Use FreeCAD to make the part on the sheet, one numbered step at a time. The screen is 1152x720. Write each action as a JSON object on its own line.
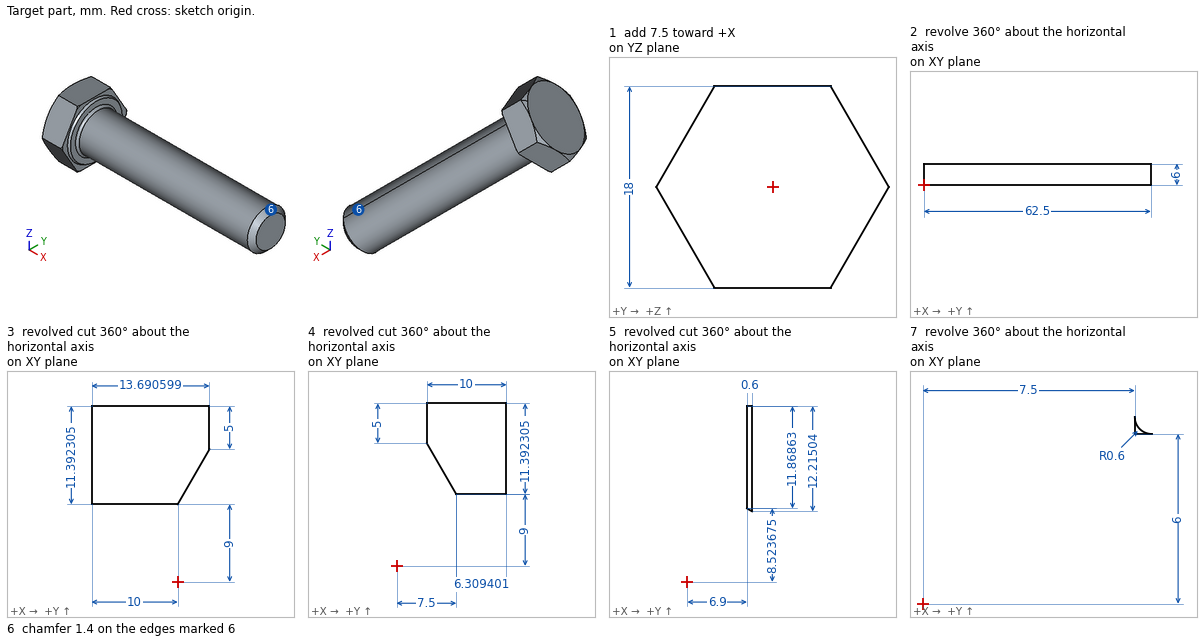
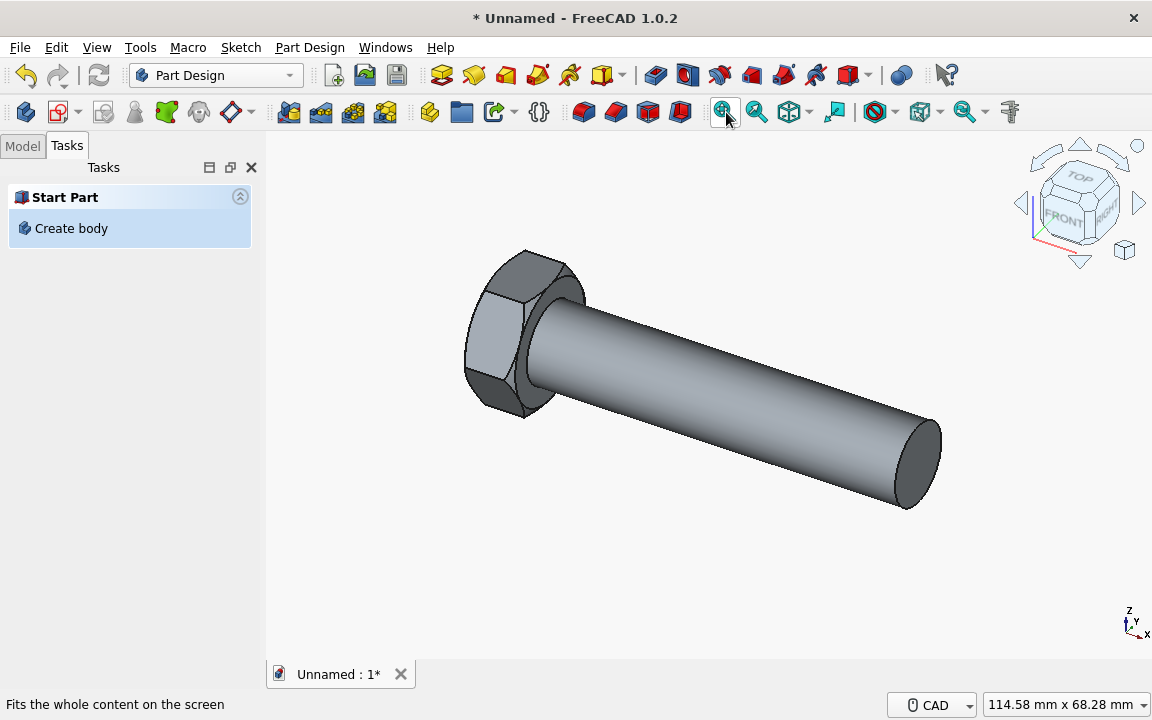
{"action": "left_click", "coordinate": [58, 112]}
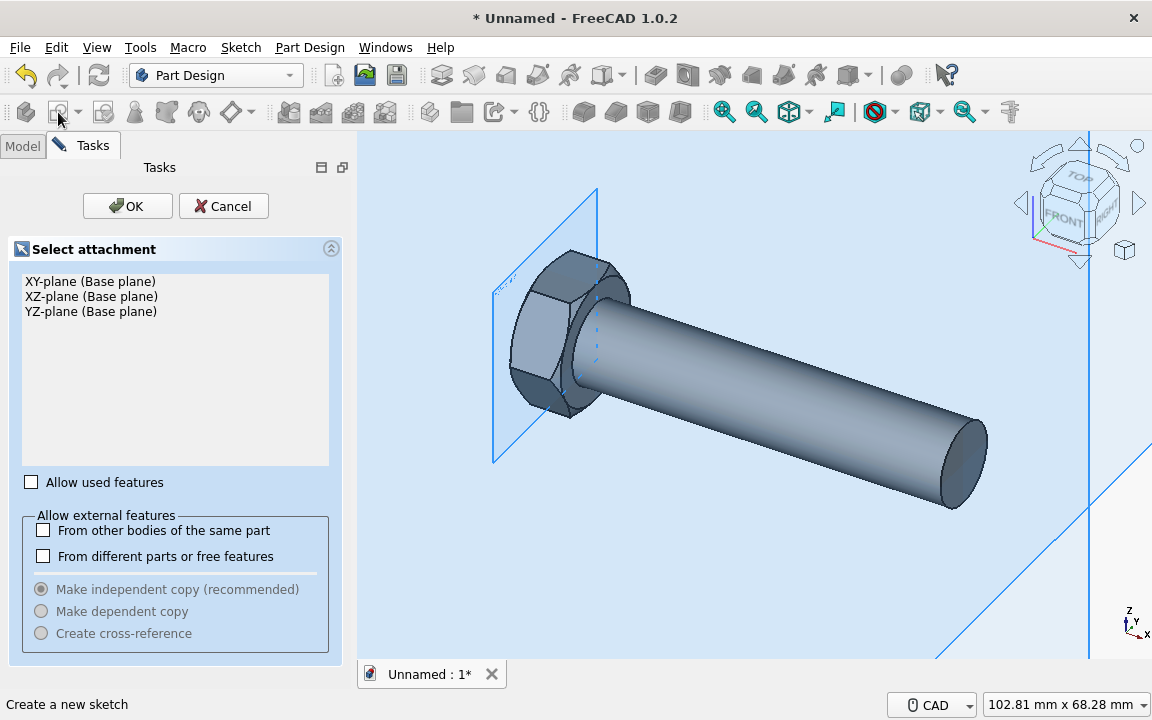
{"action": "left_click", "coordinate": [82, 282]}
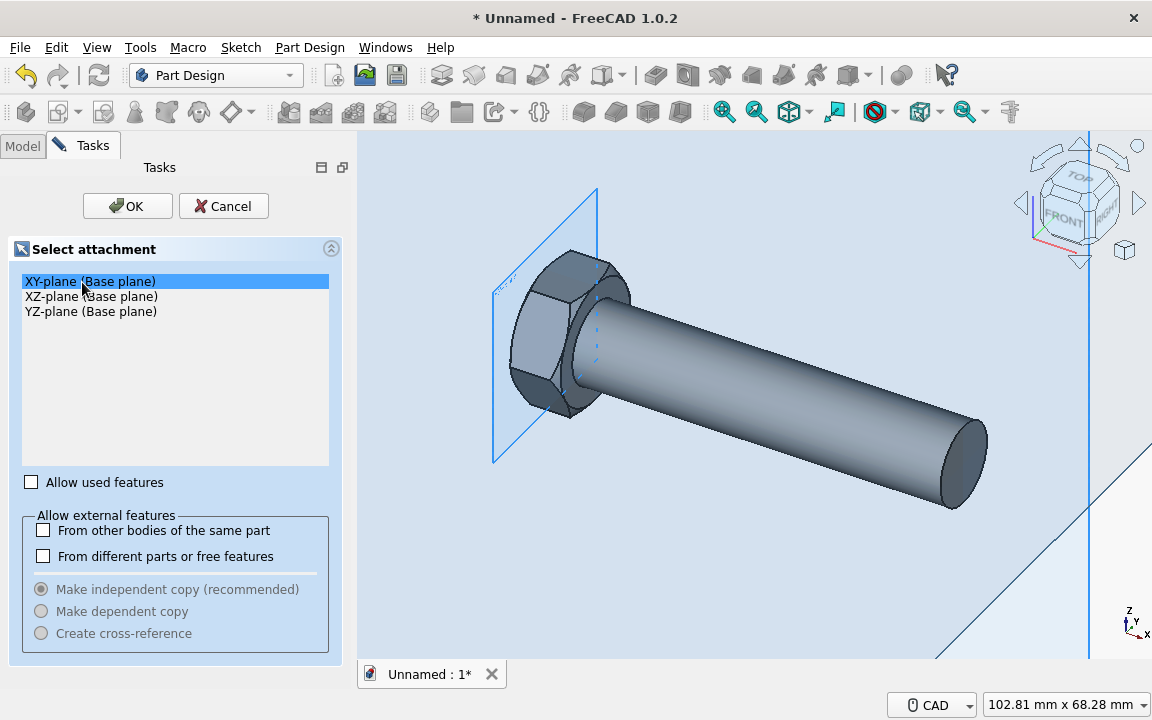
{"action": "left_click", "coordinate": [128, 206]}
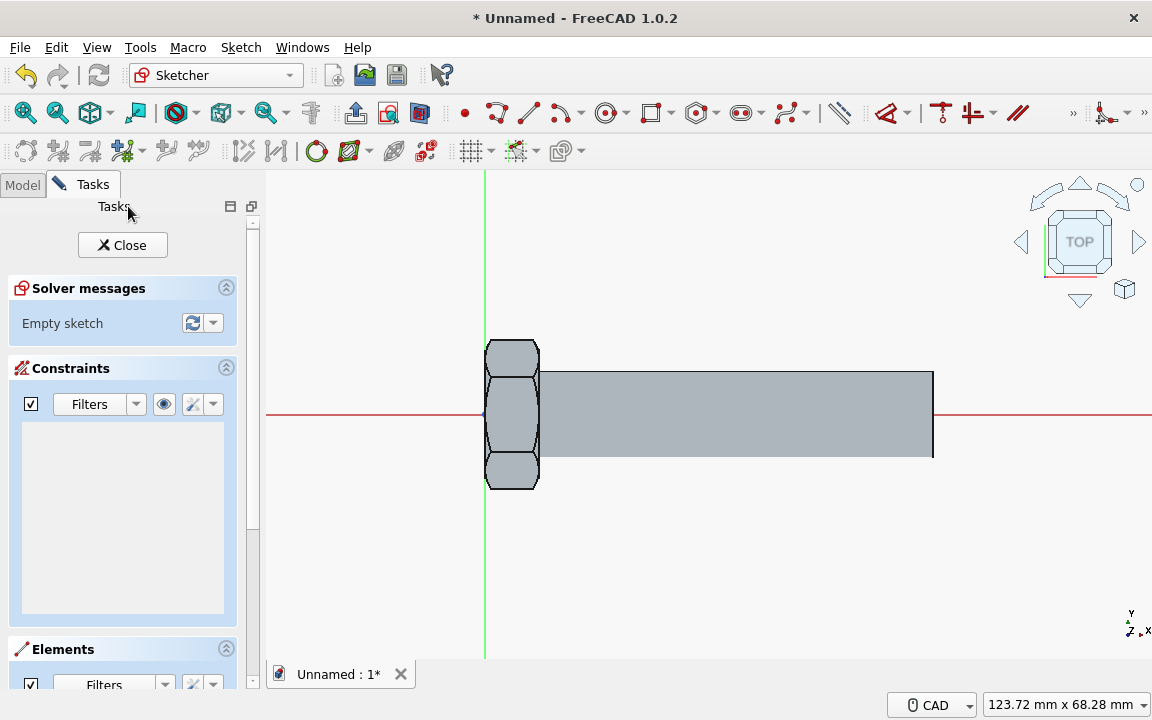
{"action": "key", "text": "q s"}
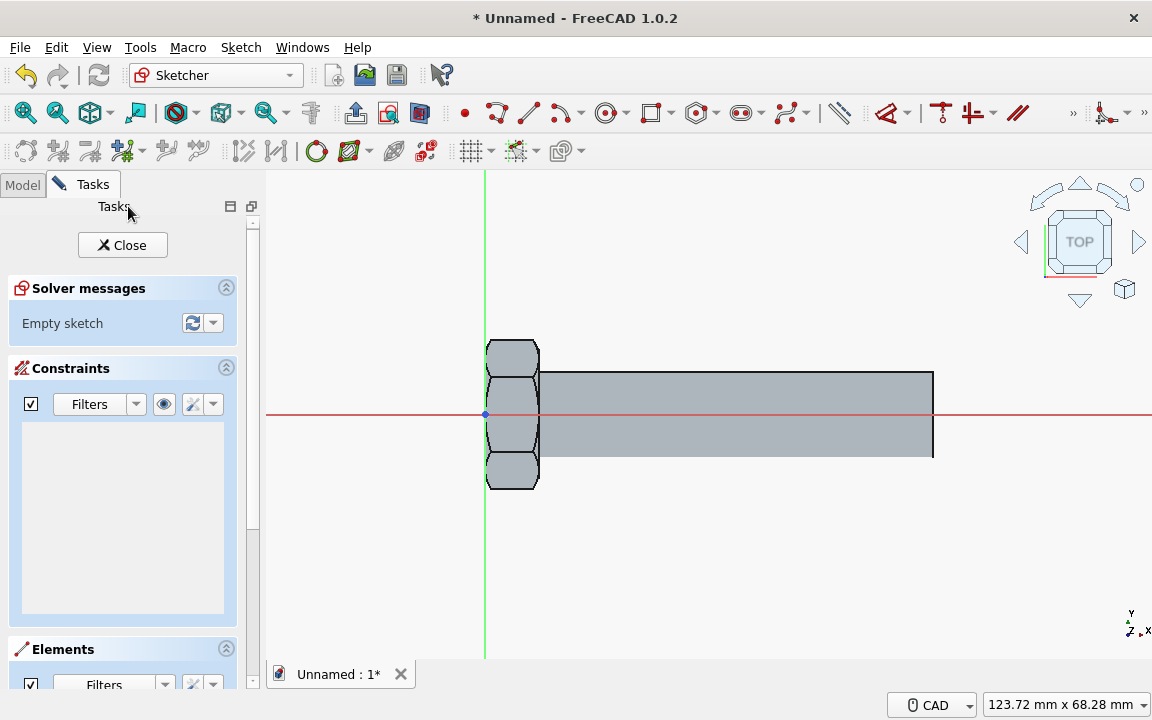
{"action": "scroll", "coordinate": [407, 282], "scroll_direction": "up", "scroll_amount": 4}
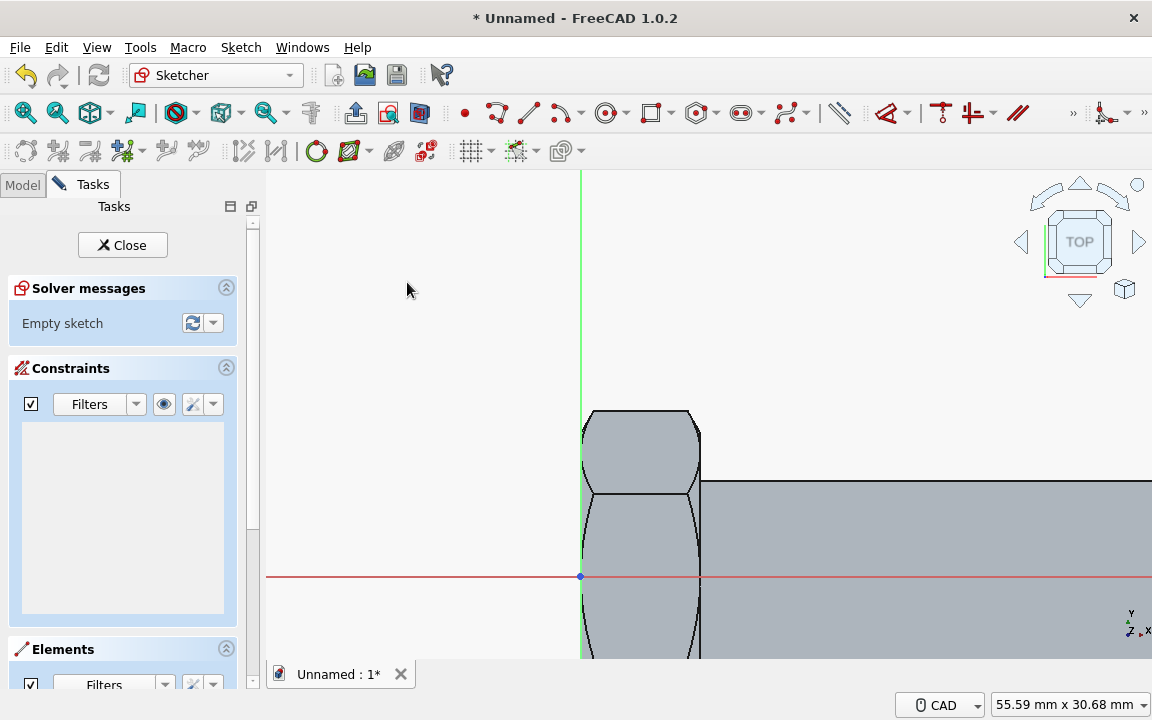
{"action": "key", "text": "g m"}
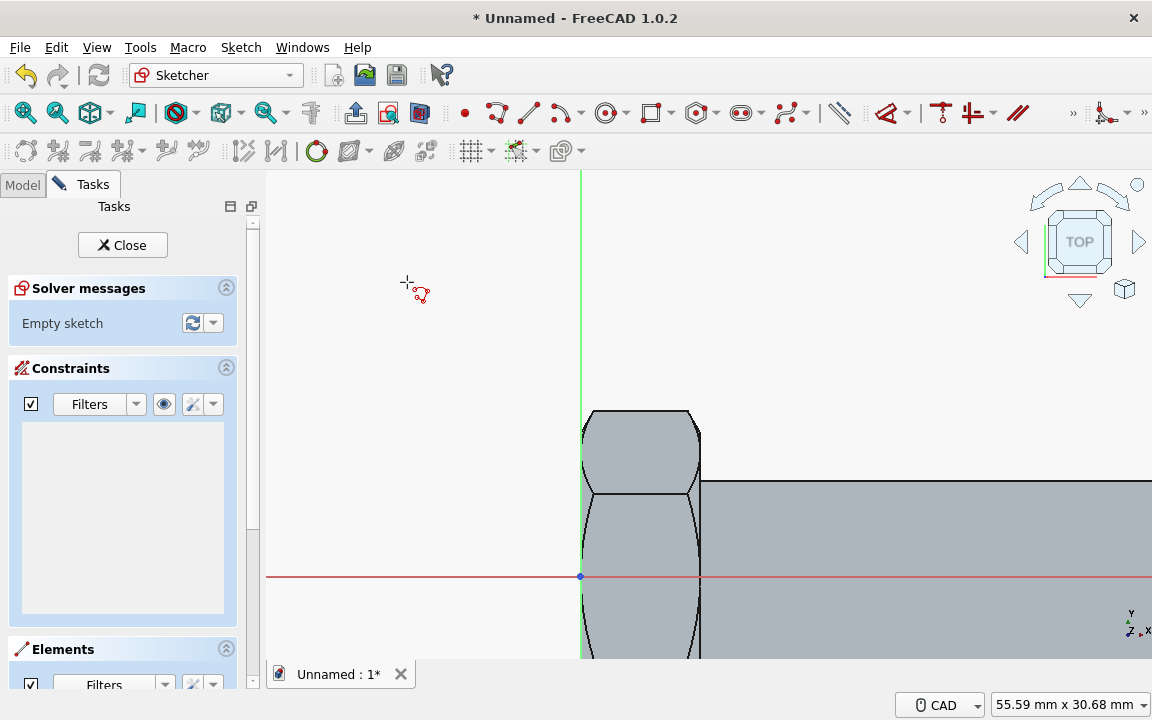
{"action": "left_click", "coordinate": [691, 441]}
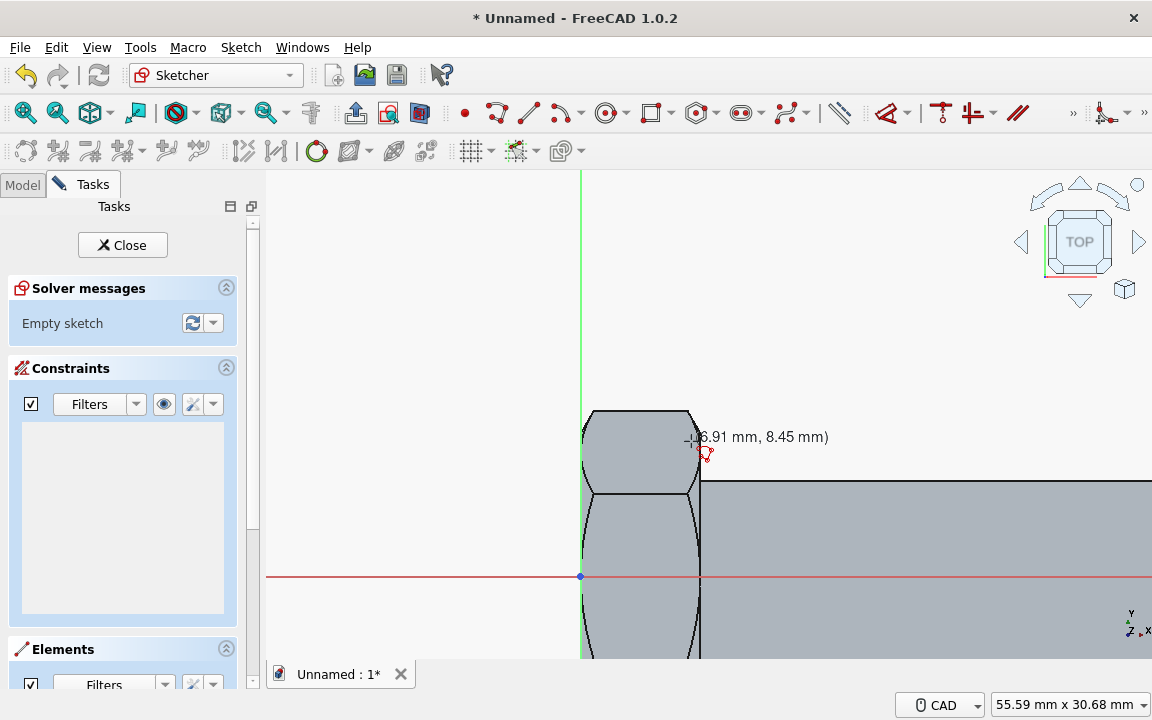
{"action": "scroll", "coordinate": [700, 446], "scroll_direction": "up", "scroll_amount": 2}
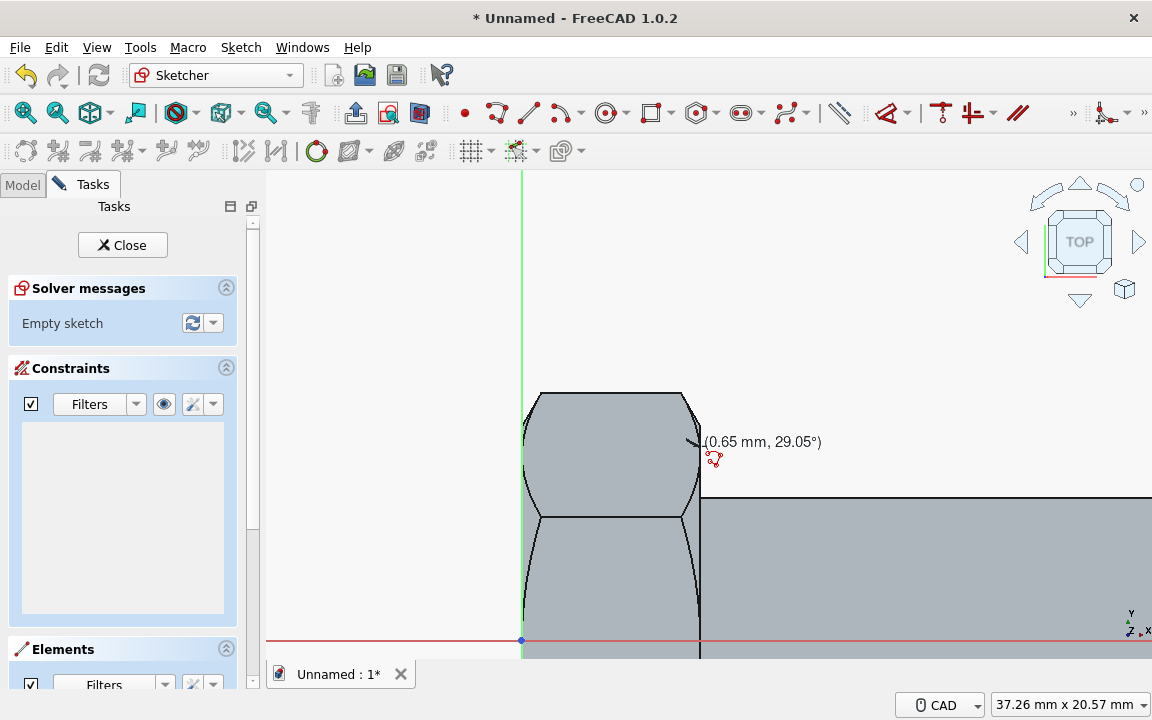
{"action": "left_click", "coordinate": [700, 446]}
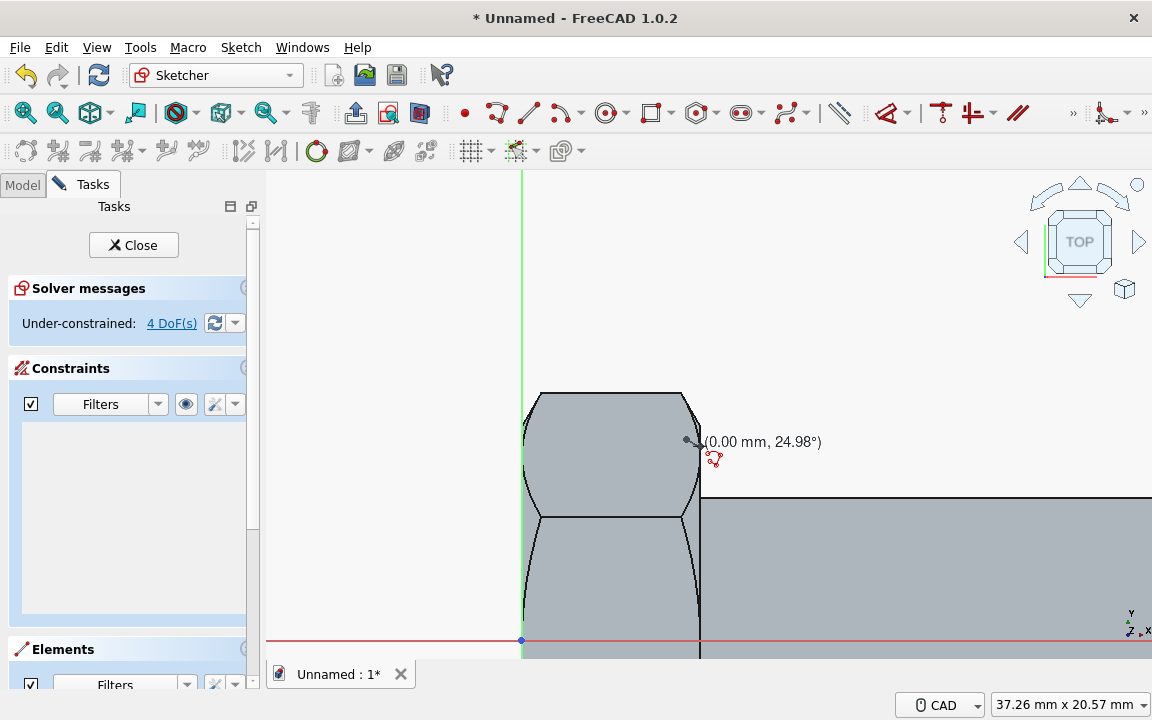
{"action": "scroll", "coordinate": [700, 448], "scroll_direction": "down", "scroll_amount": 2}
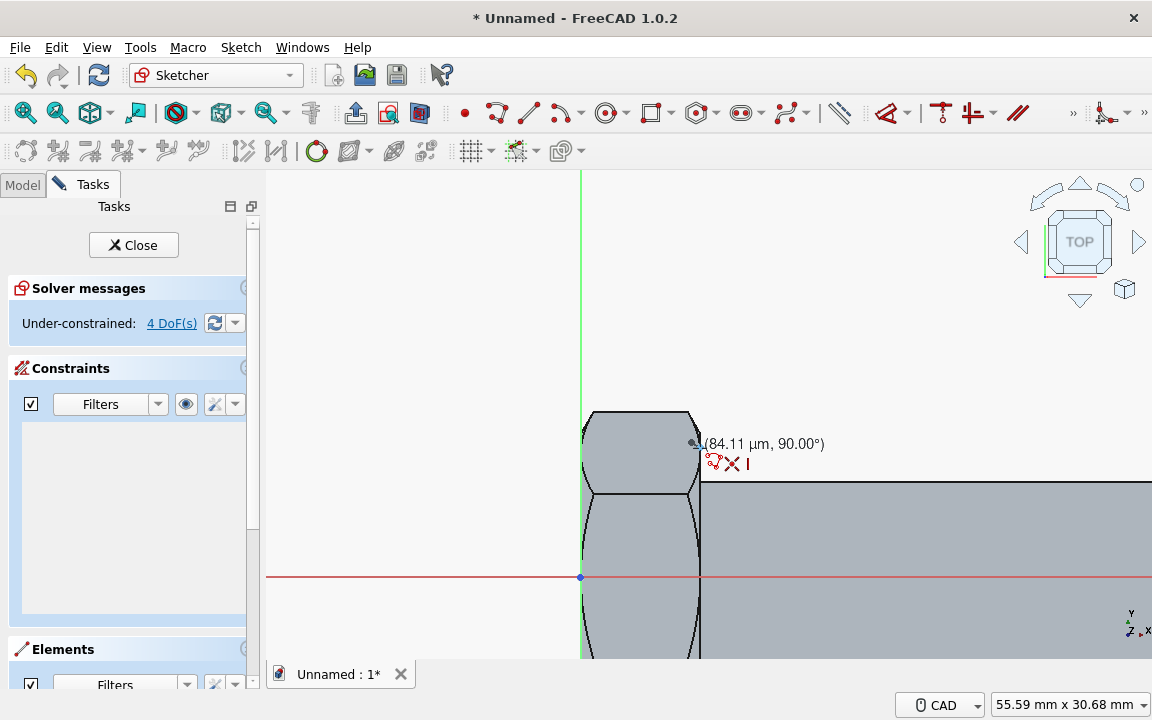
{"action": "left_click", "coordinate": [700, 252]}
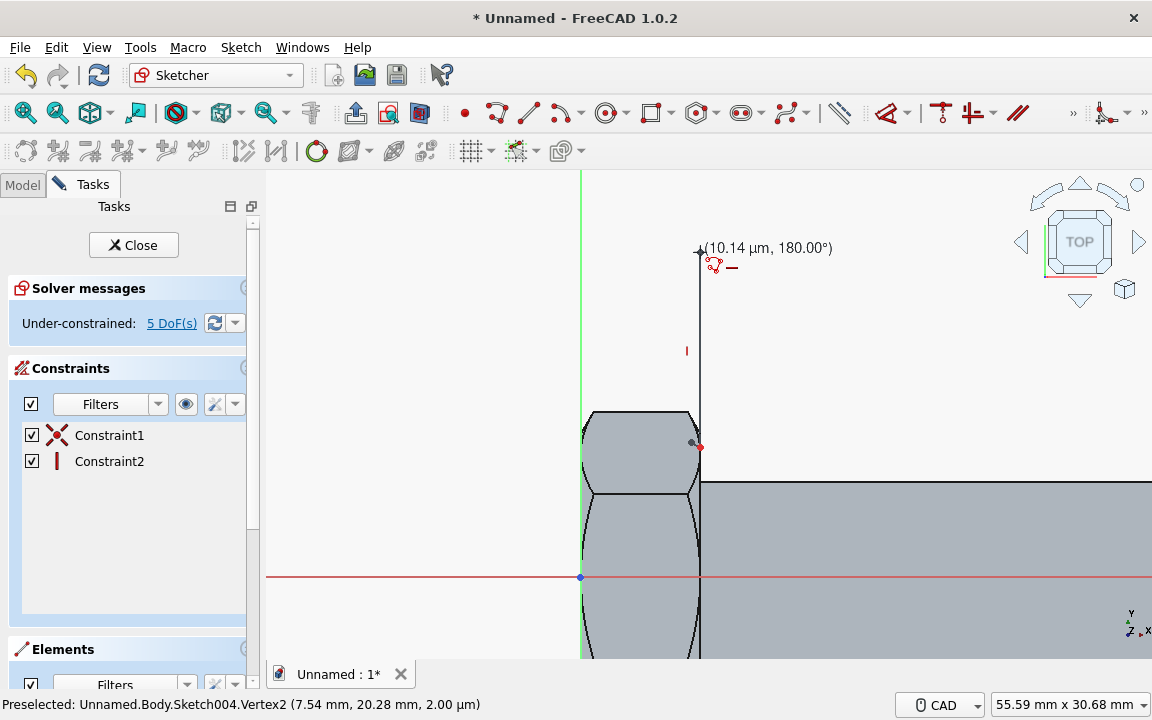
{"action": "scroll", "coordinate": [691, 252], "scroll_direction": "up", "scroll_amount": 3}